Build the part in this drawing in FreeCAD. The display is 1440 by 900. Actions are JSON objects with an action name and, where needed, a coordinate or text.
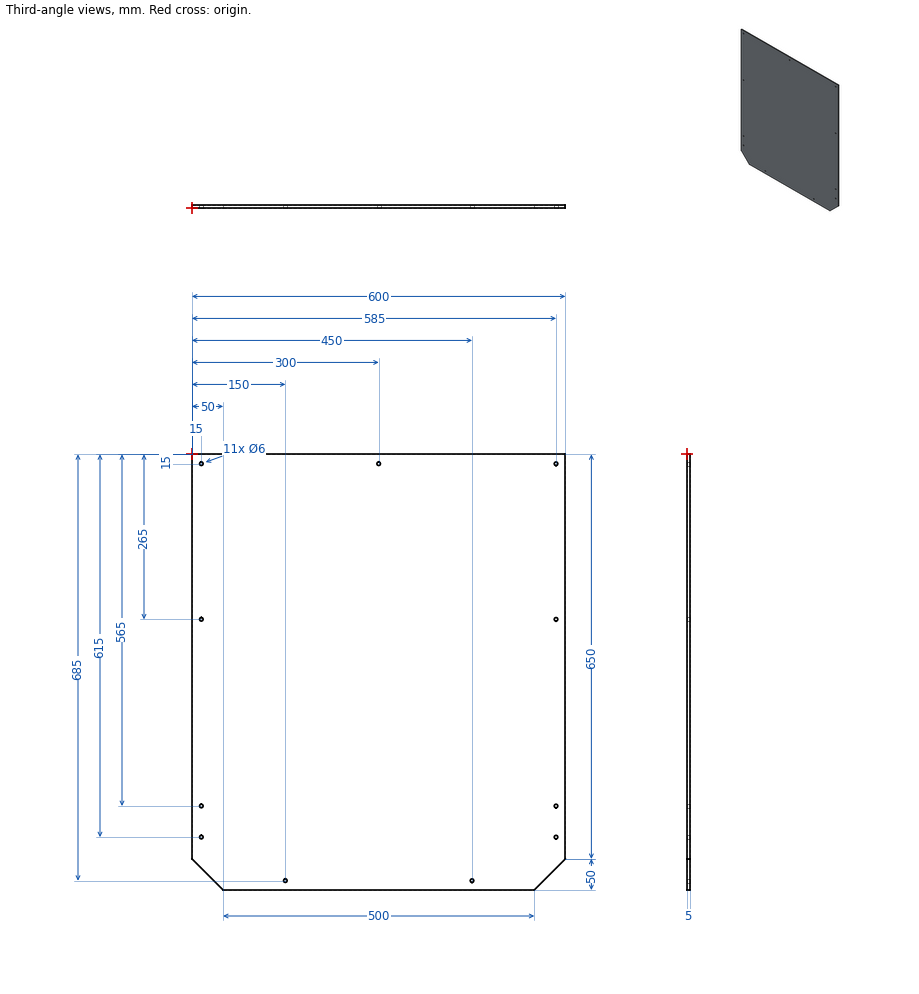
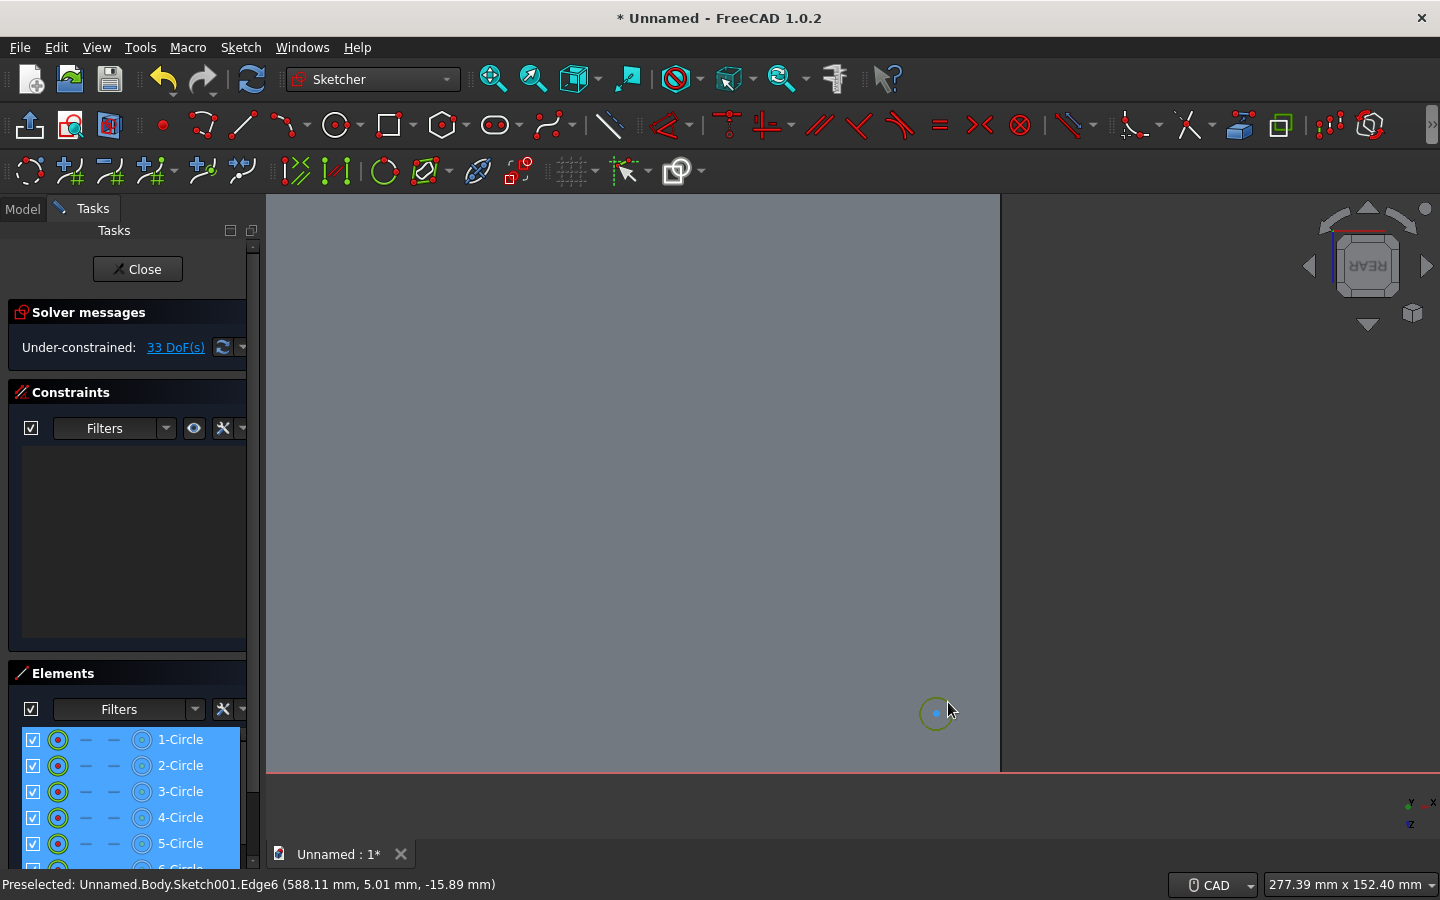
{"action": "scroll", "coordinate": [953, 704], "scroll_direction": "down", "scroll_amount": 10}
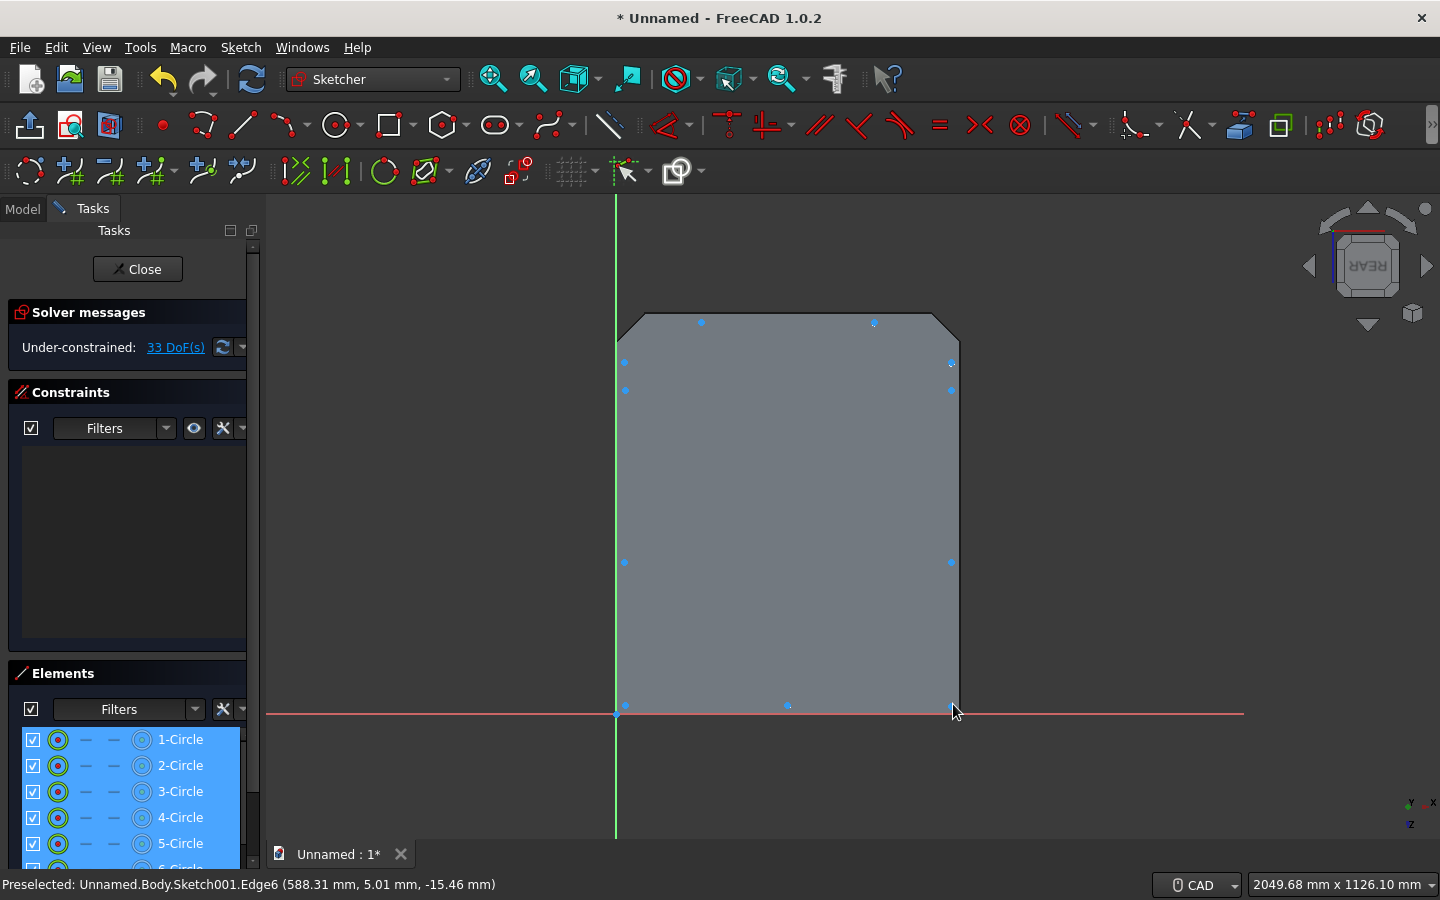
{"action": "scroll", "coordinate": [953, 561], "scroll_direction": "up", "scroll_amount": 9}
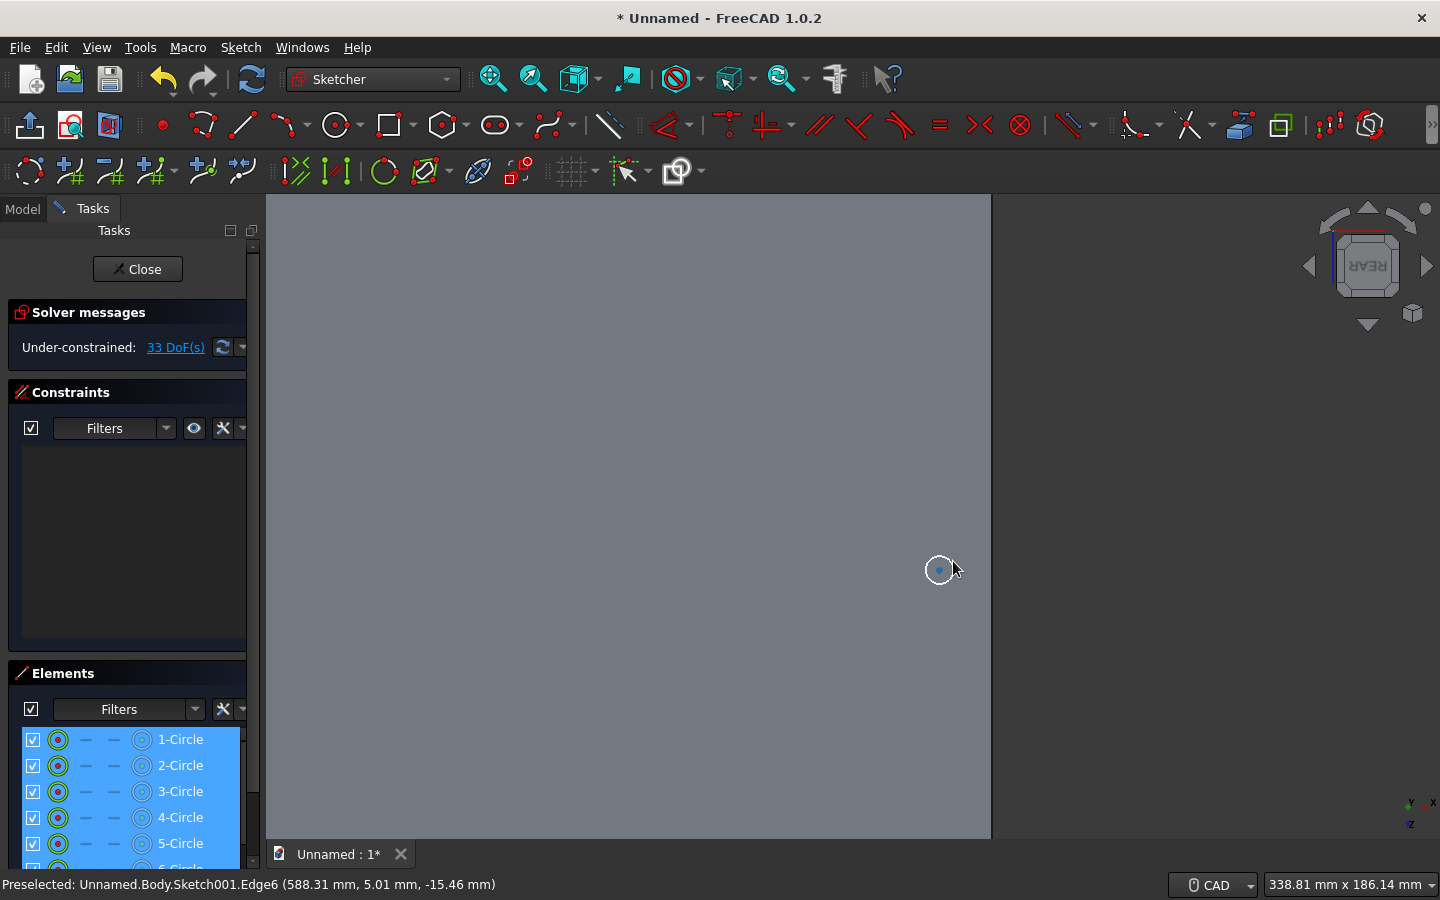
{"action": "left_click", "coordinate": [949, 560]}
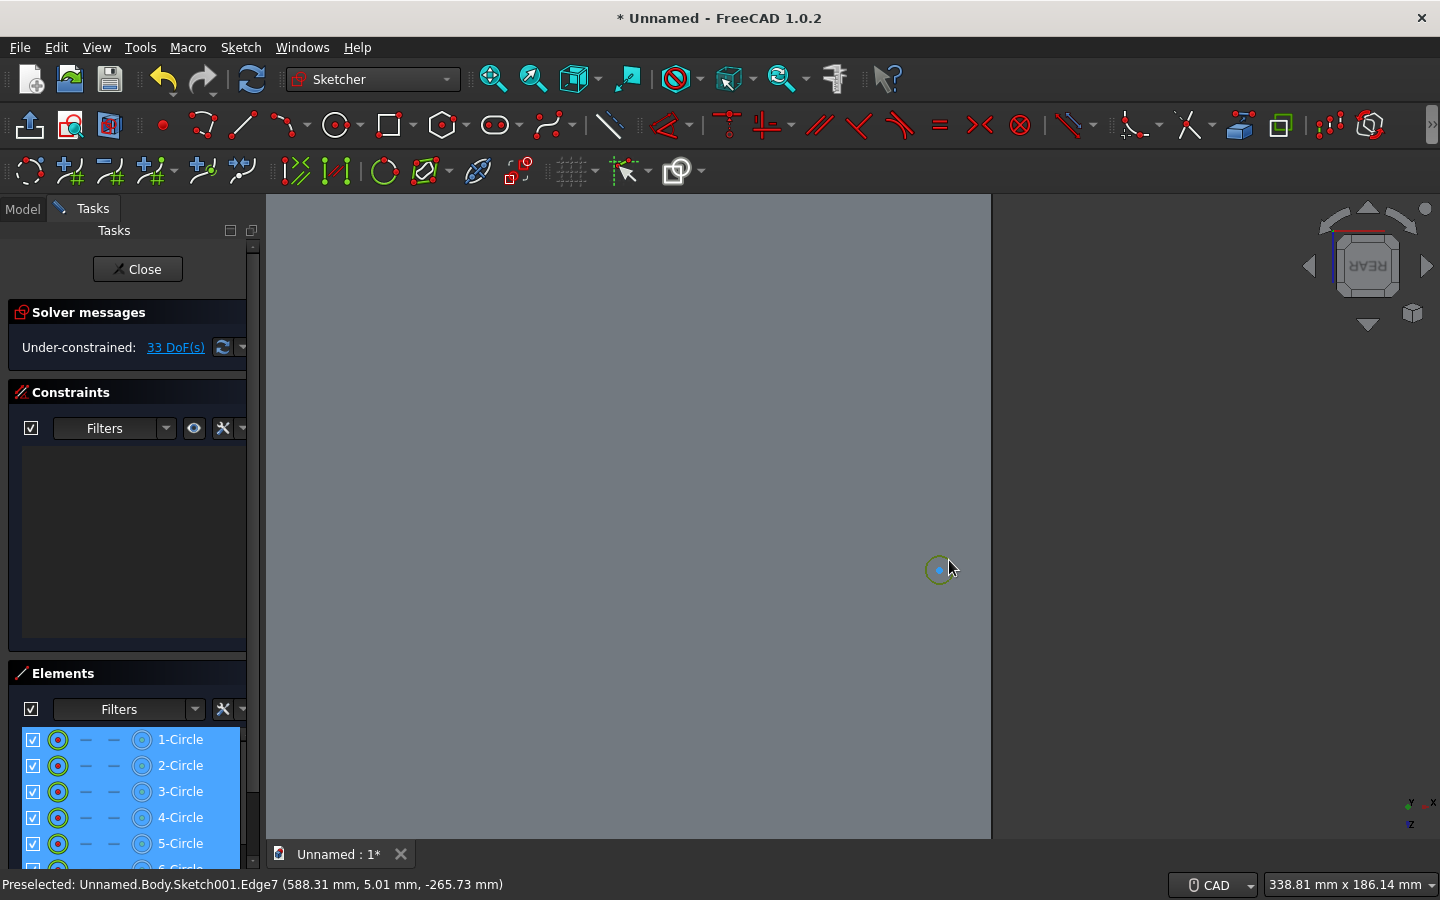
{"action": "scroll", "coordinate": [953, 561], "scroll_direction": "down", "scroll_amount": 9}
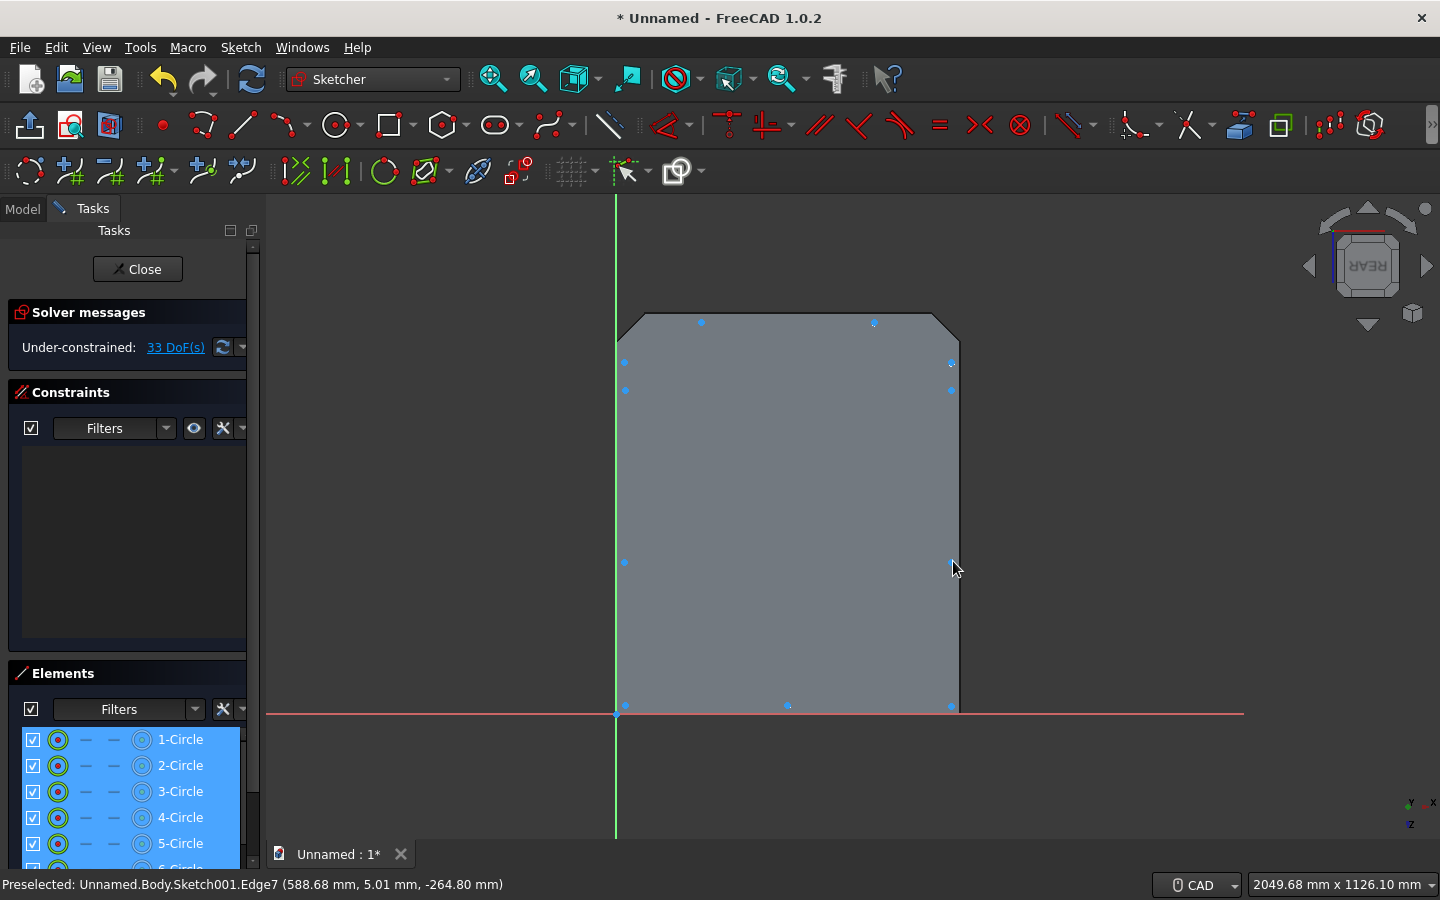
{"action": "scroll", "coordinate": [953, 389], "scroll_direction": "up", "scroll_amount": 10}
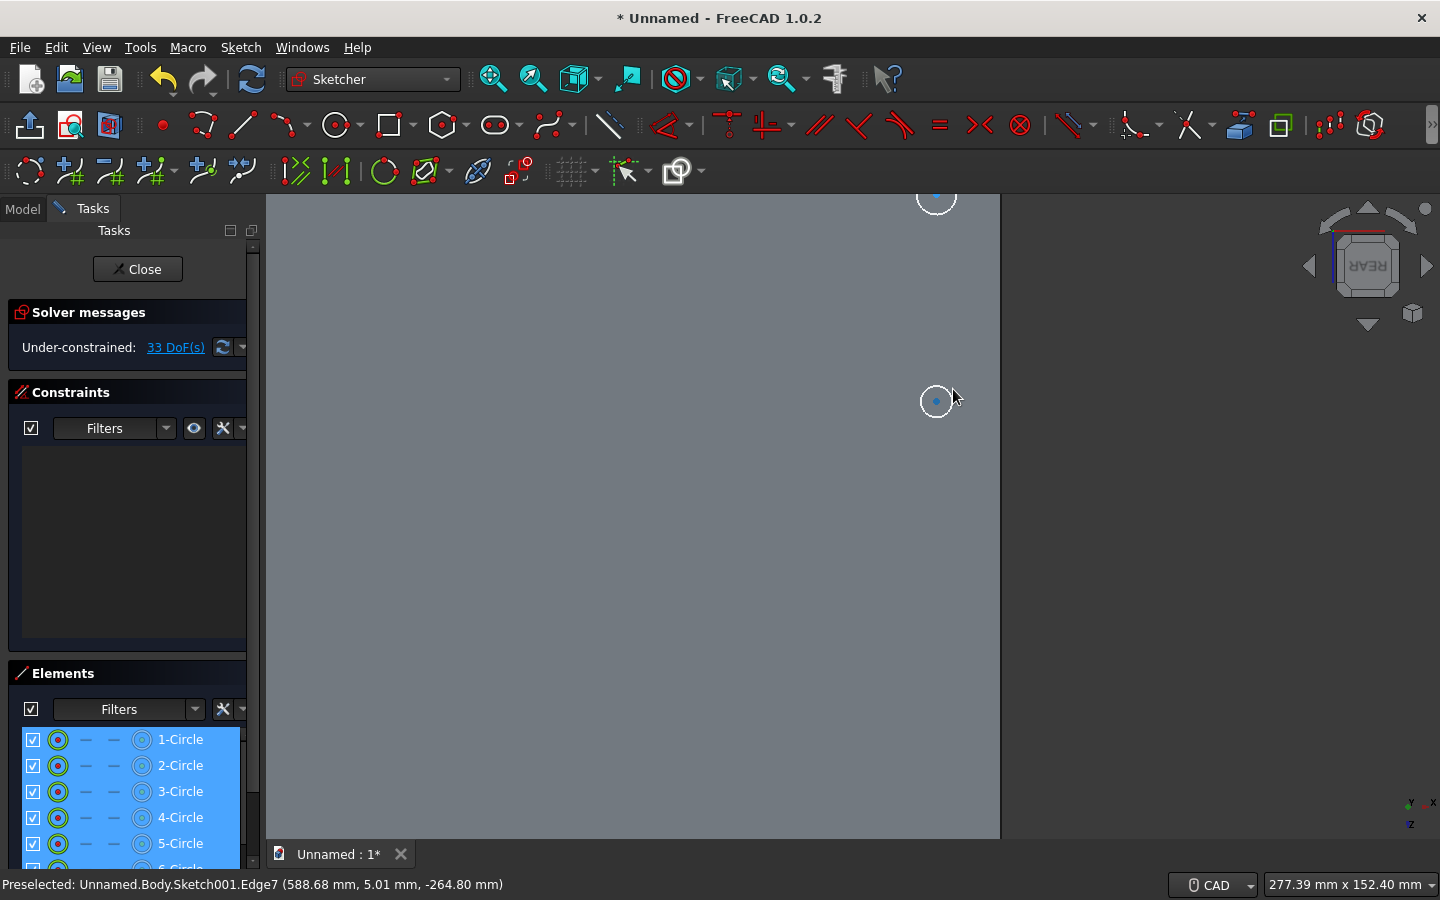
{"action": "left_click", "coordinate": [948, 391]}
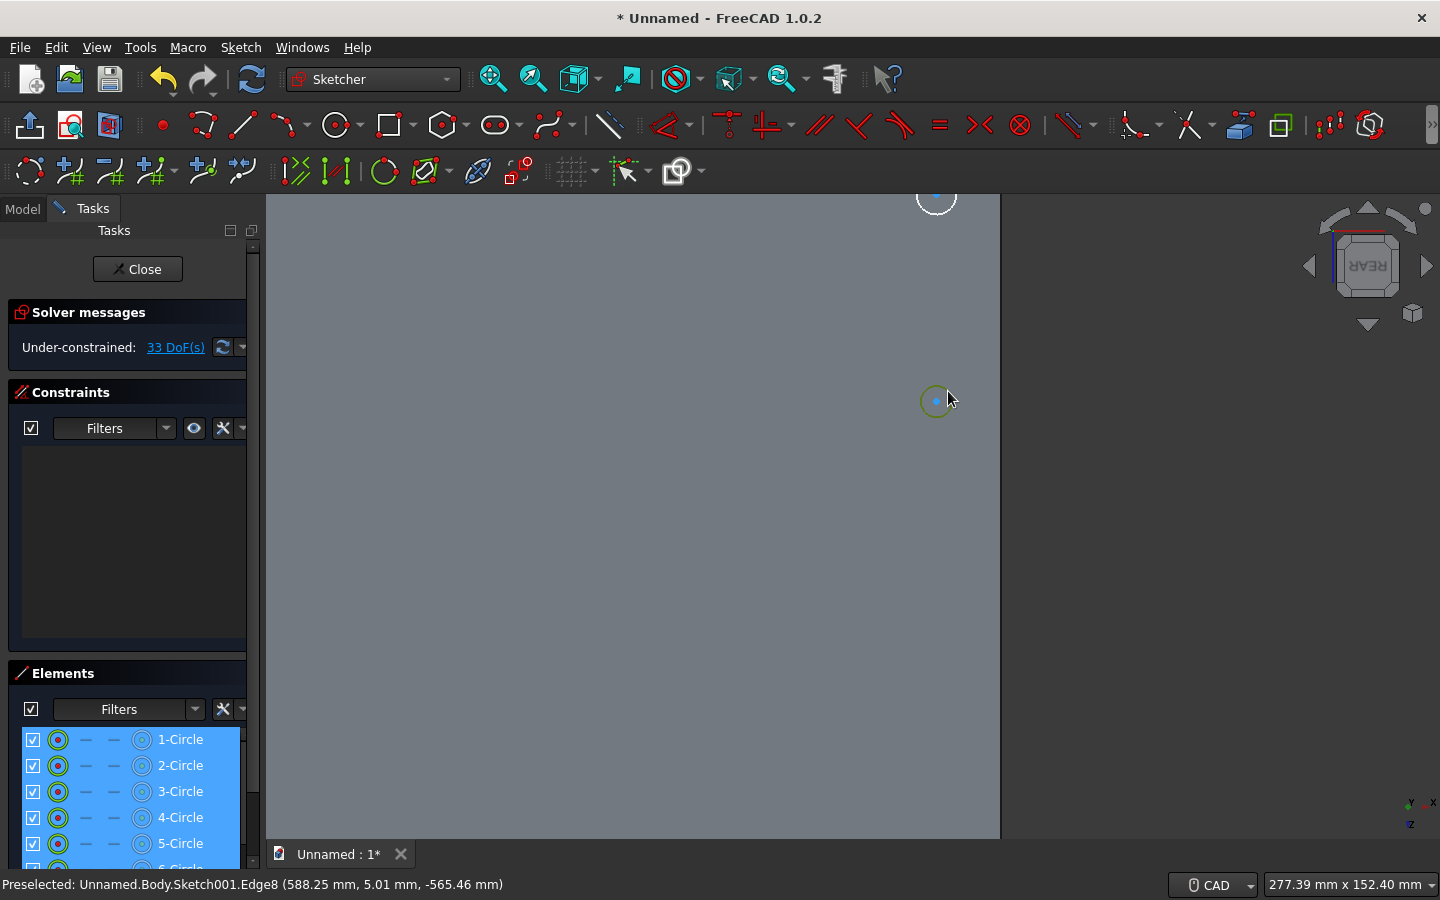
{"action": "scroll", "coordinate": [953, 389], "scroll_direction": "down", "scroll_amount": 10}